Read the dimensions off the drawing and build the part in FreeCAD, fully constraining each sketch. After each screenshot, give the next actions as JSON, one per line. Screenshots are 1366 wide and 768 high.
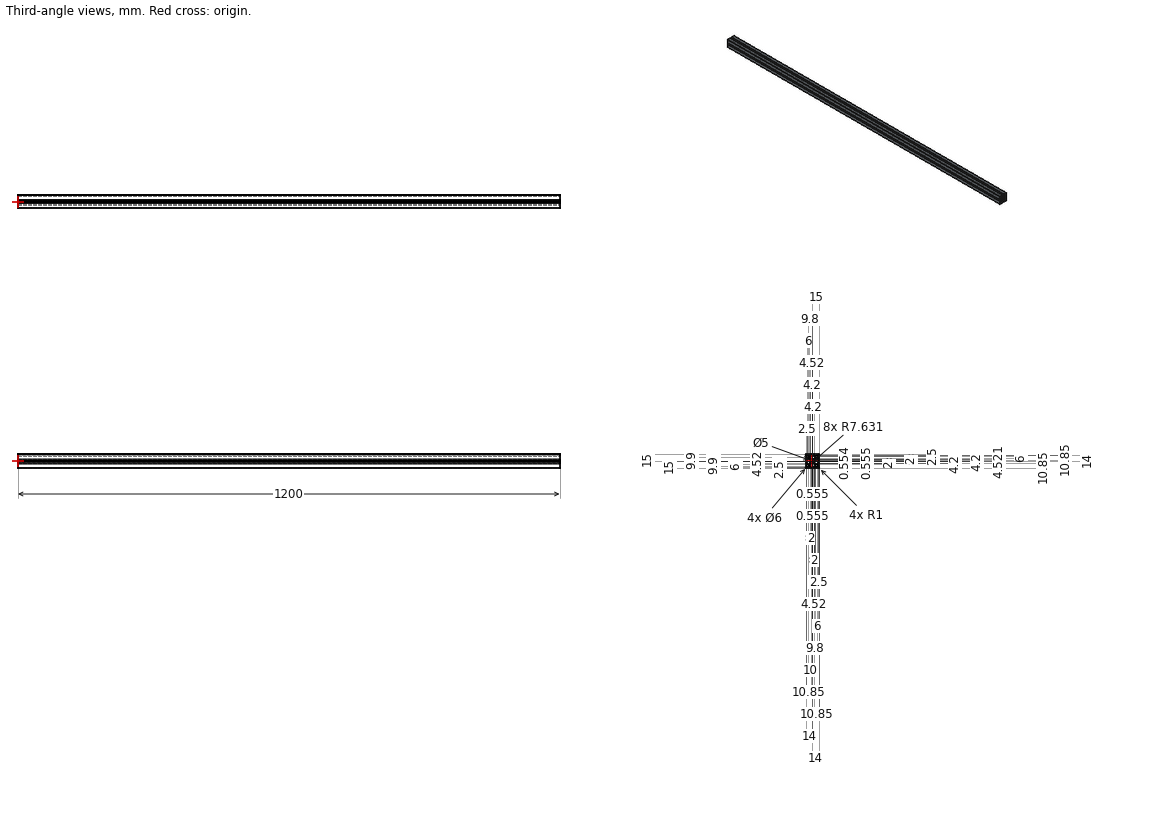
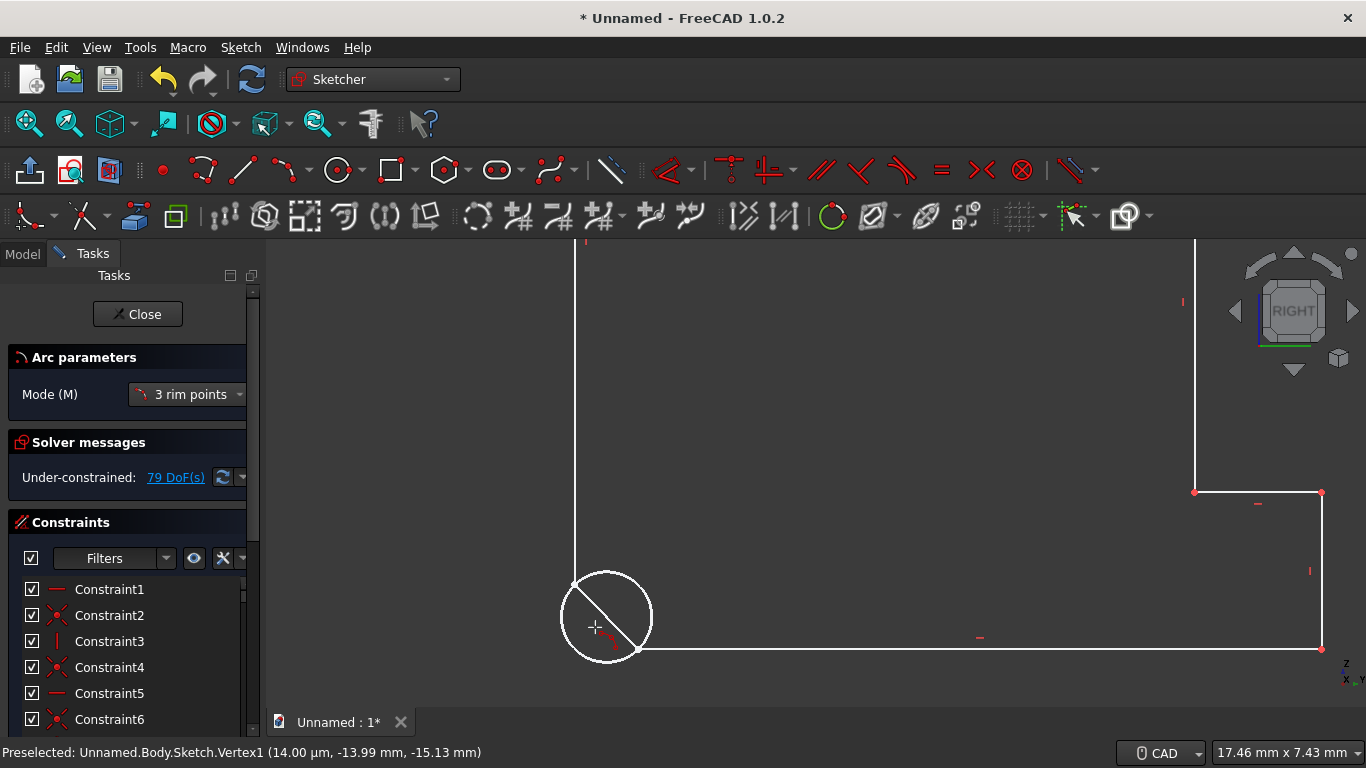
{"action": "left_click", "coordinate": [593, 623]}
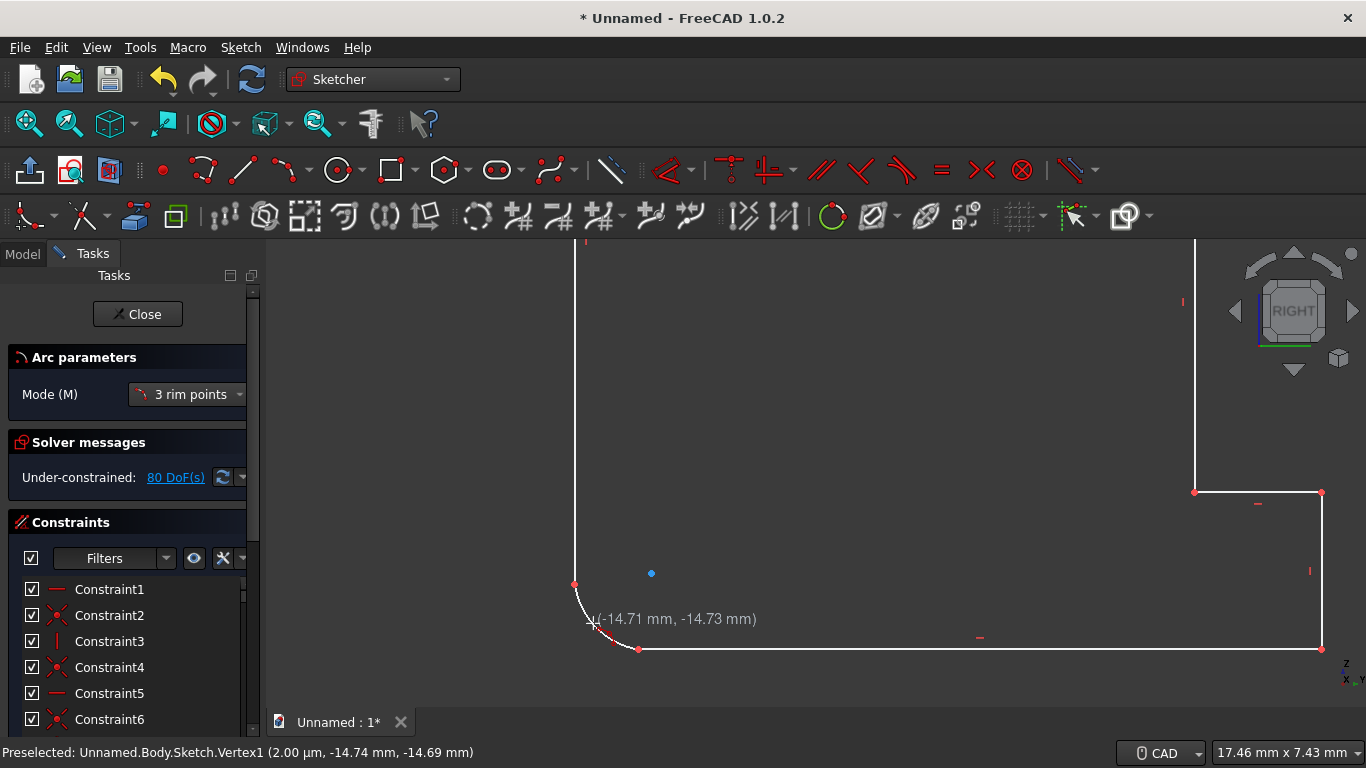
{"action": "left_click", "coordinate": [338, 170]}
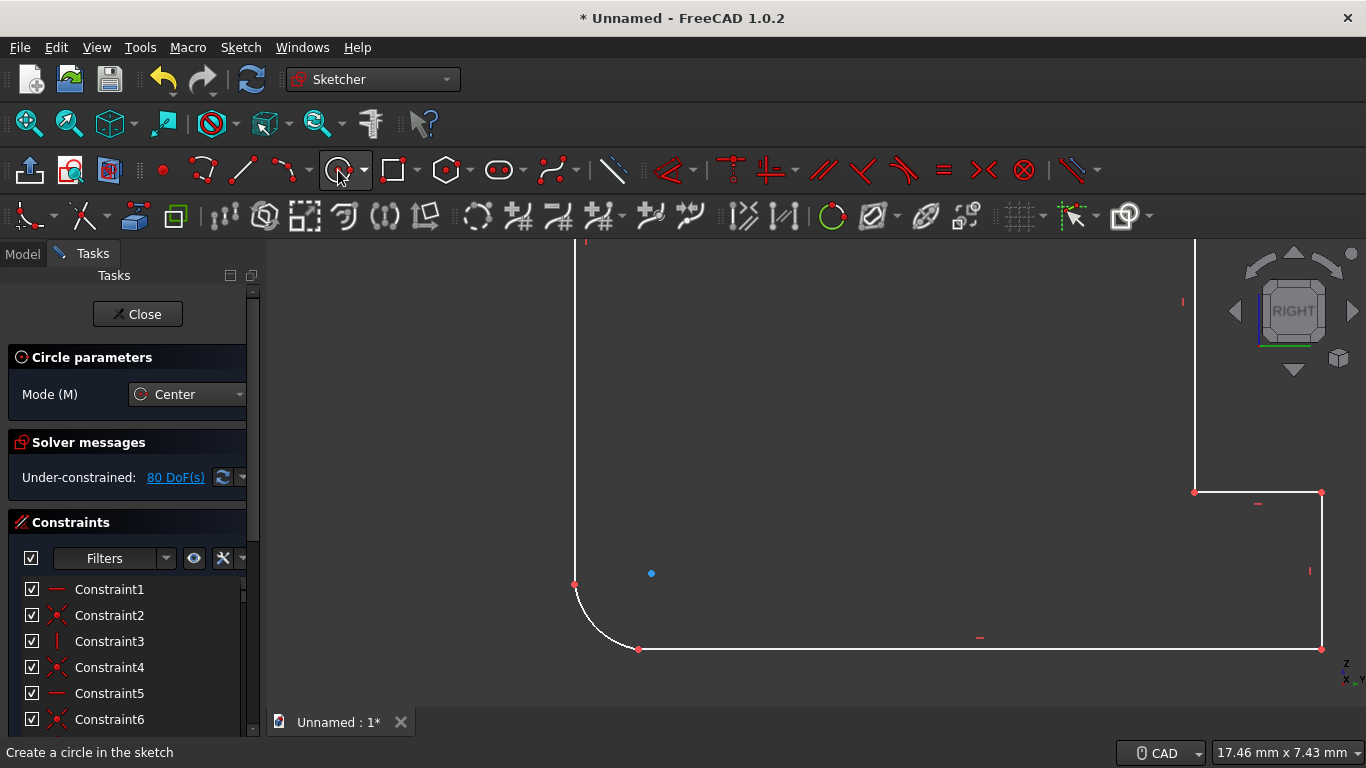
{"action": "scroll", "coordinate": [595, 627], "scroll_direction": "down", "scroll_amount": 9}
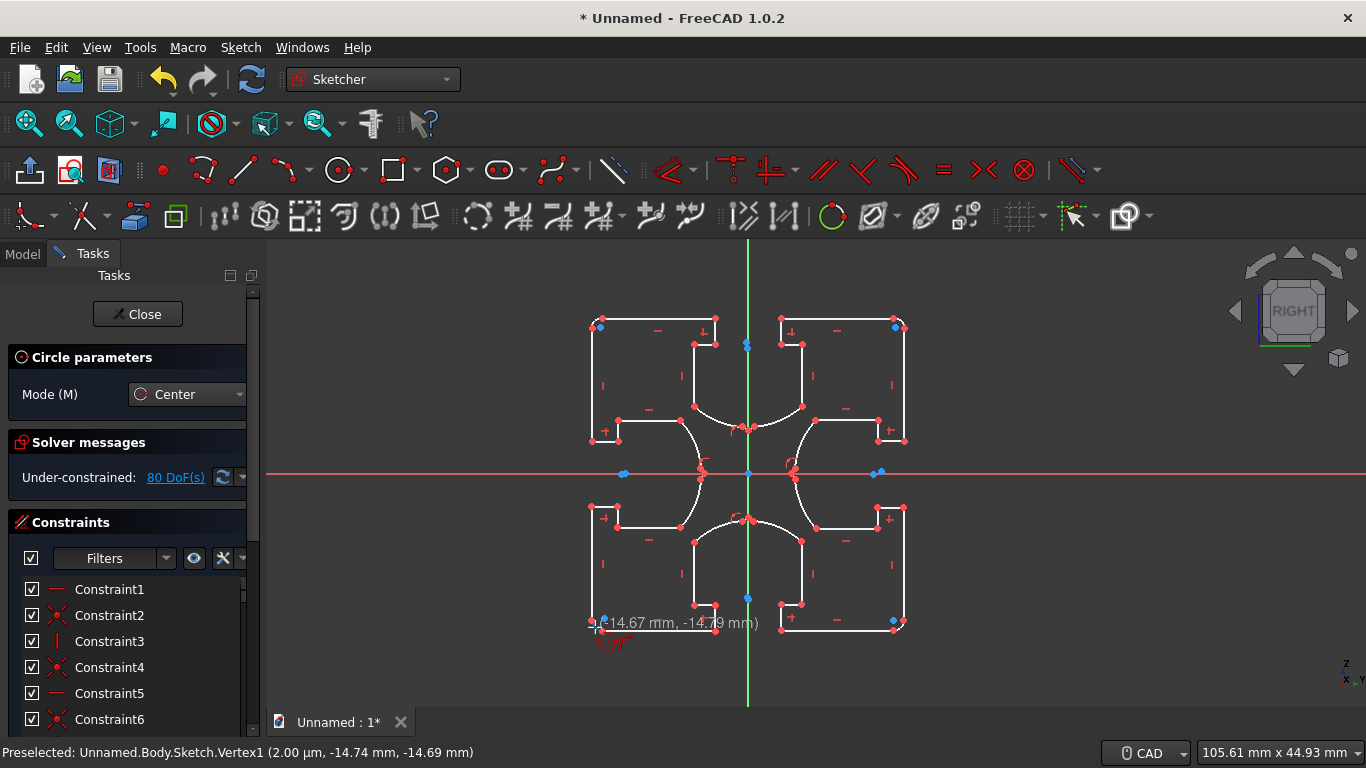
{"action": "left_click", "coordinate": [644, 577]}
{"action": "left_click", "coordinate": [666, 555]}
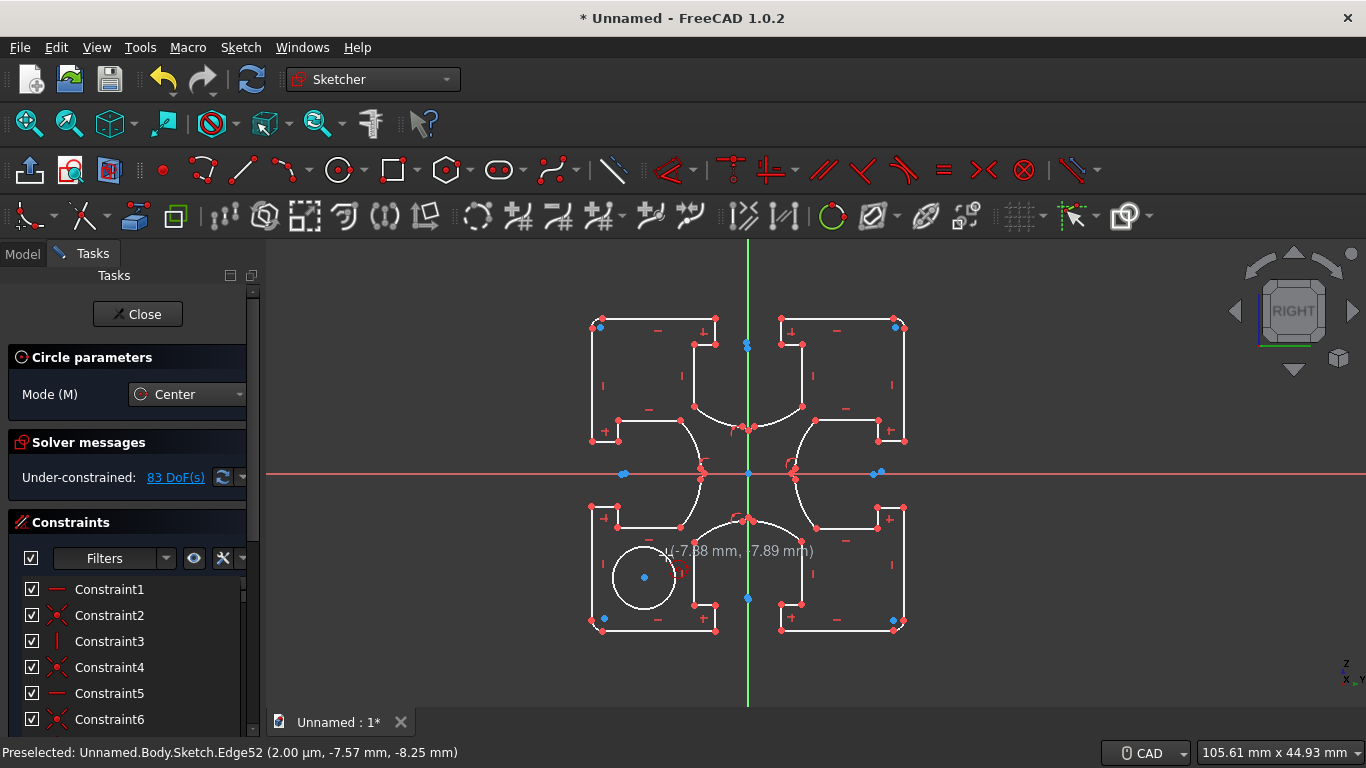
{"action": "left_click", "coordinate": [850, 577]}
{"action": "left_click", "coordinate": [872, 555]}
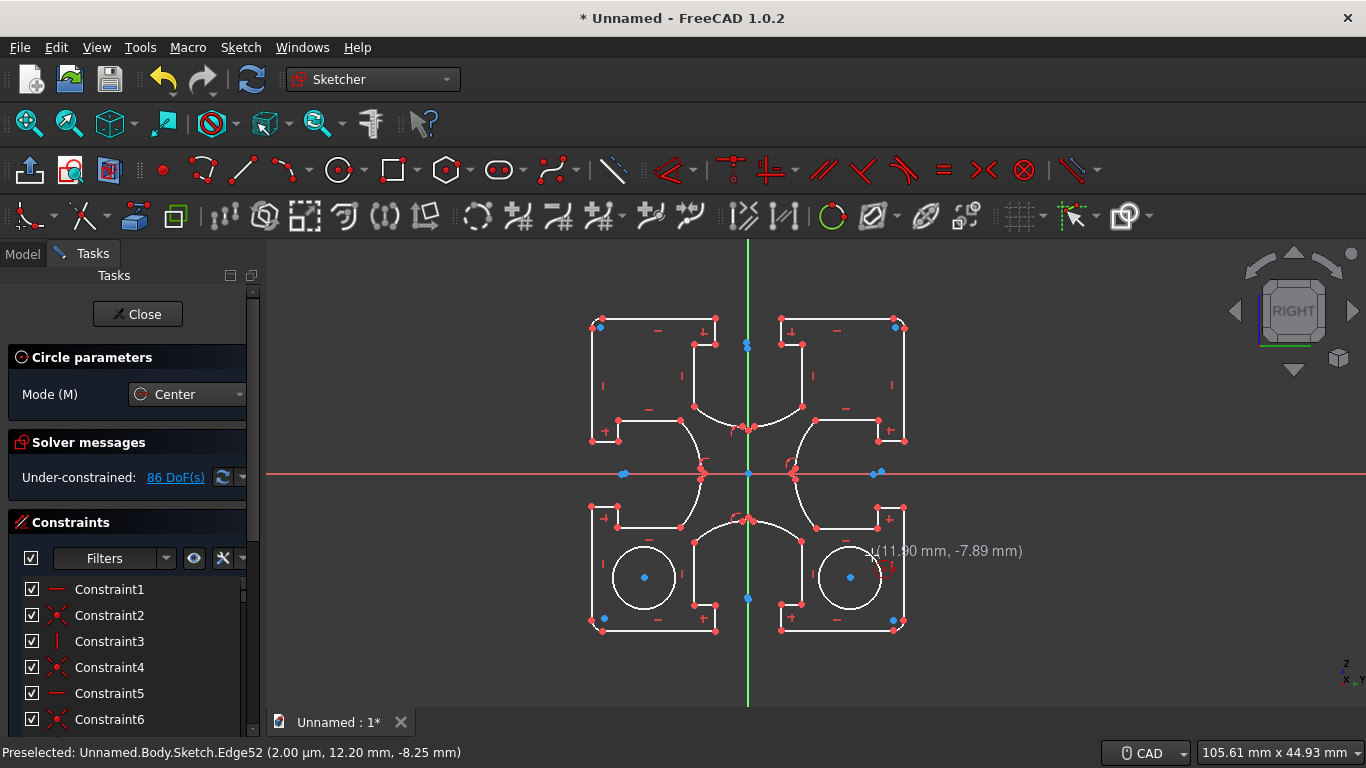
{"action": "left_click", "coordinate": [646, 371]}
{"action": "left_click", "coordinate": [668, 349]}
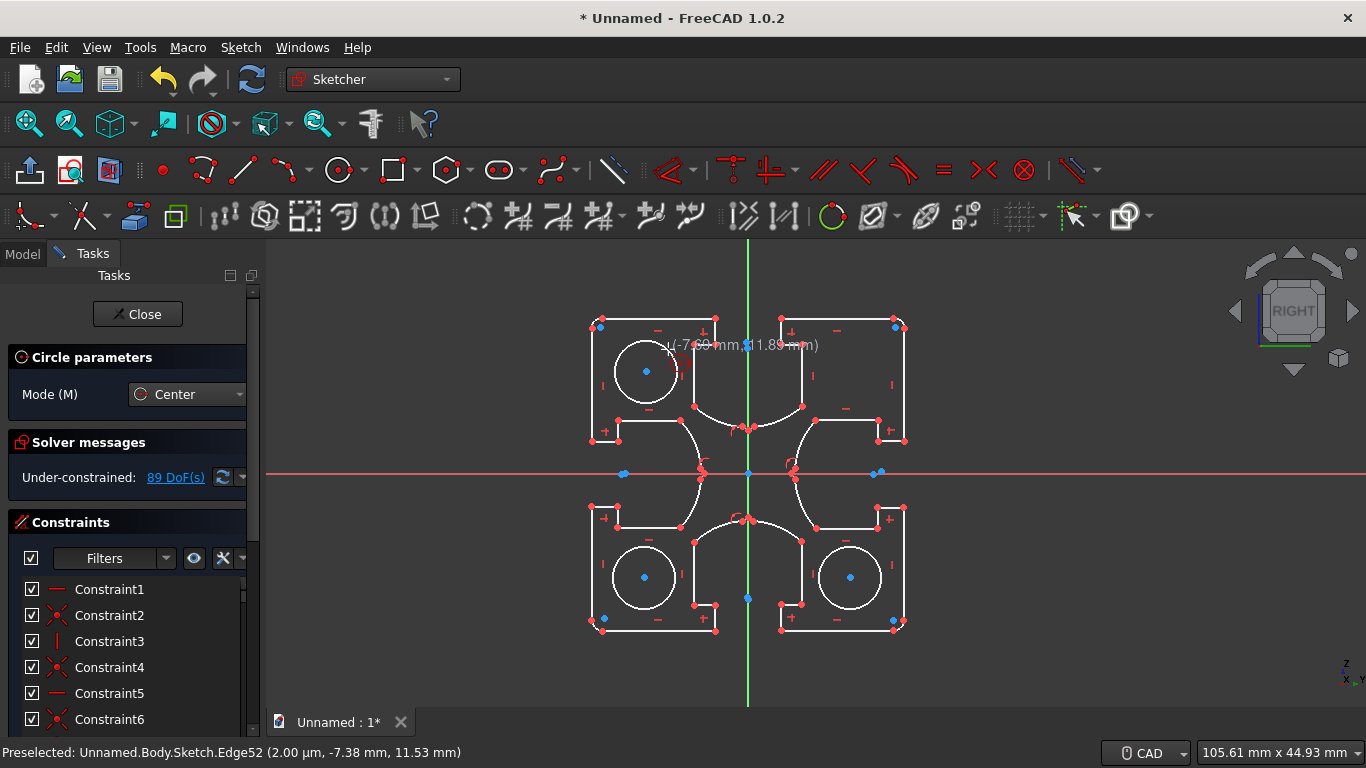
{"action": "left_click", "coordinate": [748, 474]}
{"action": "left_click", "coordinate": [767, 455]}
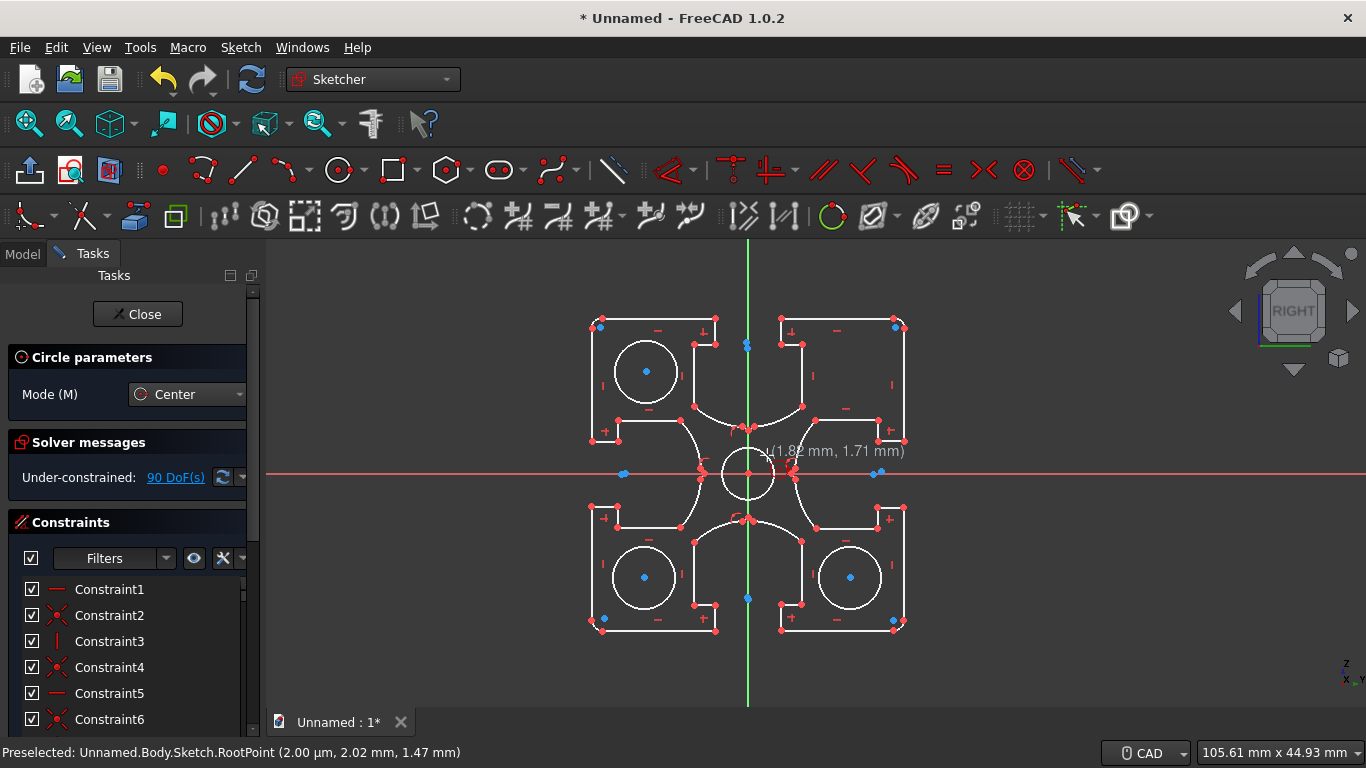
{"action": "left_click", "coordinate": [850, 371]}
{"action": "left_click", "coordinate": [872, 349]}
{"action": "key", "text": "Escape"}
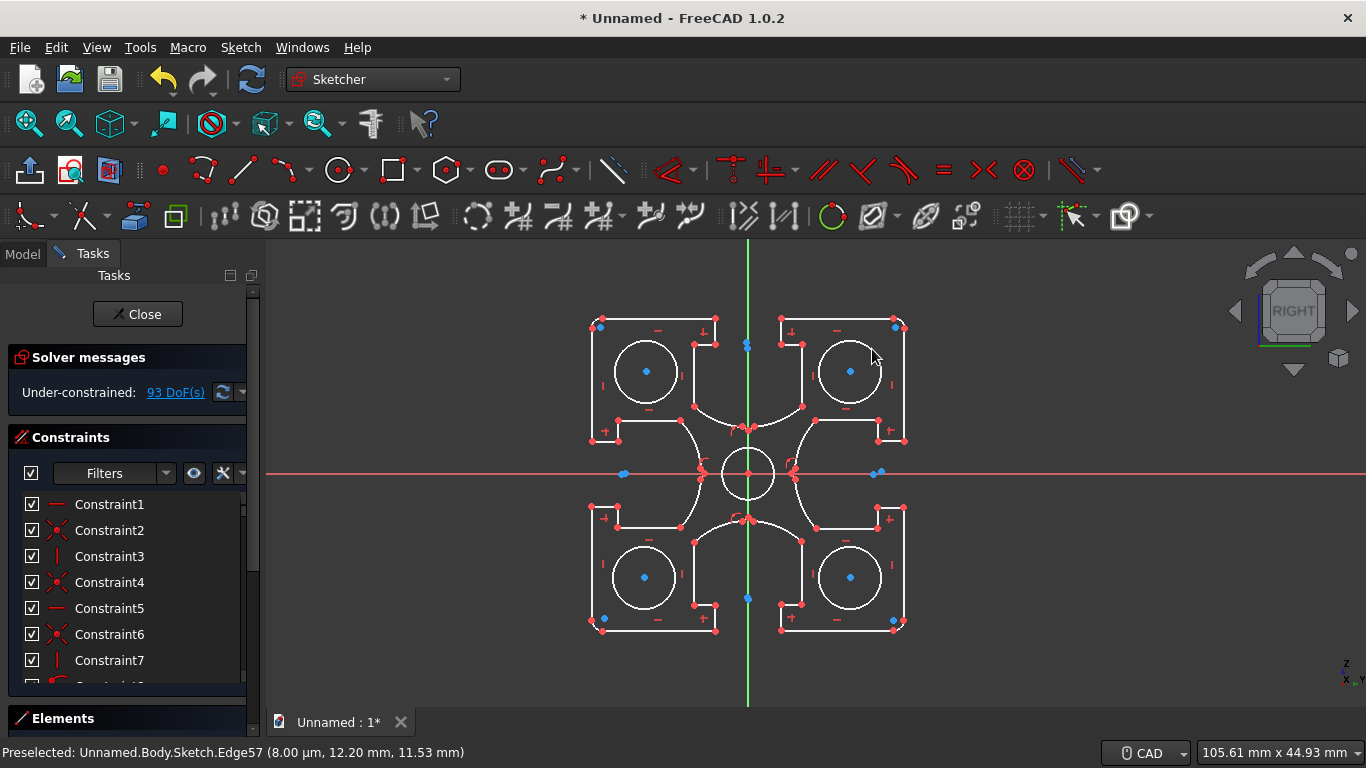
{"action": "left_click", "coordinate": [636, 631]}